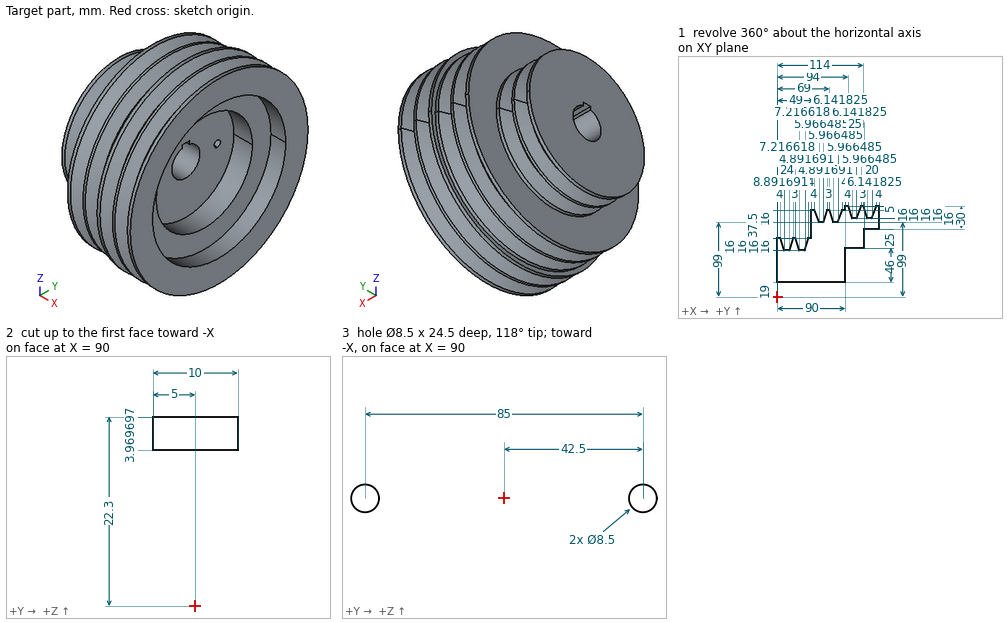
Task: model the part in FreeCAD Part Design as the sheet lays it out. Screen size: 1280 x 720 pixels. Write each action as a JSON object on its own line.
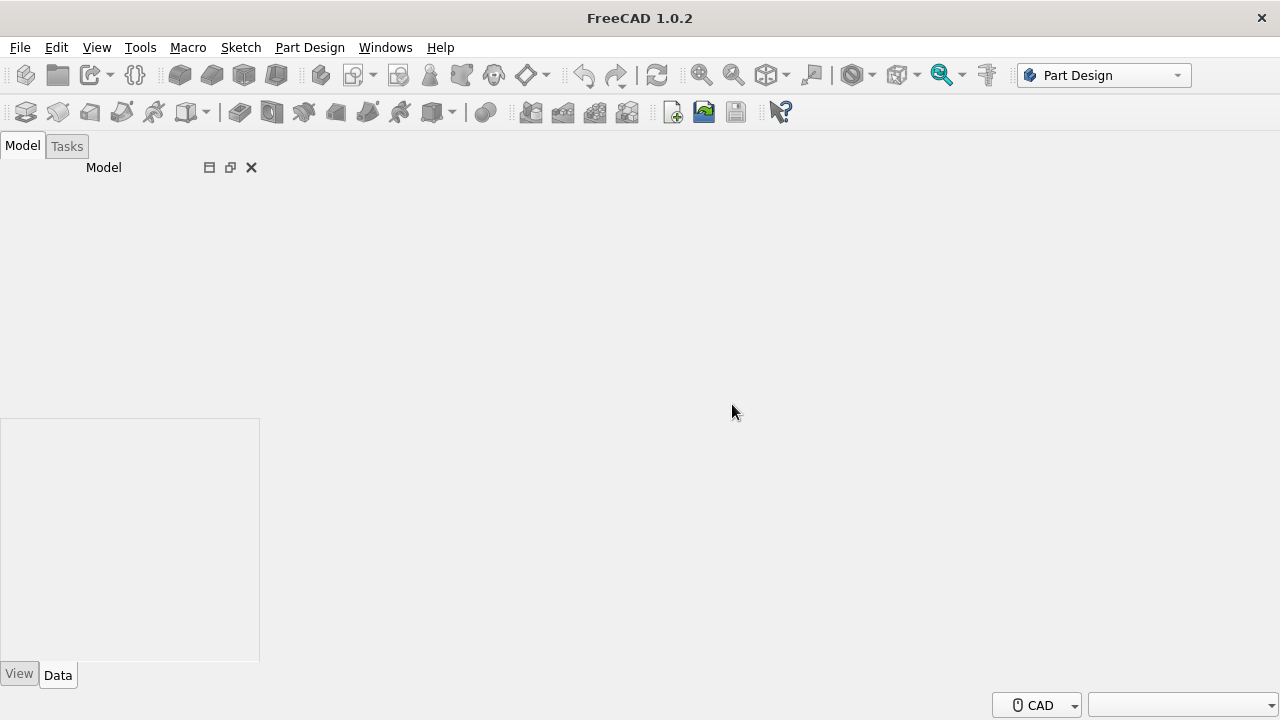
{"action": "key", "text": "ctrl+n"}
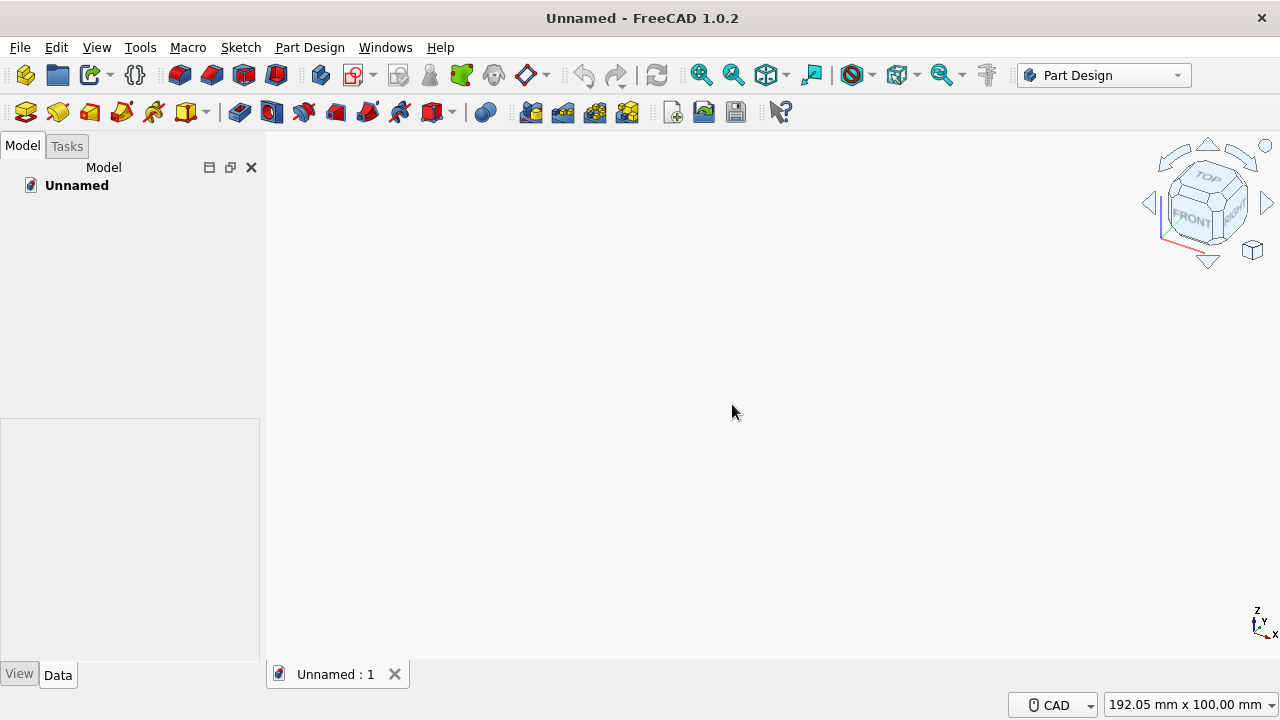
{"action": "left_click", "coordinate": [354, 76]}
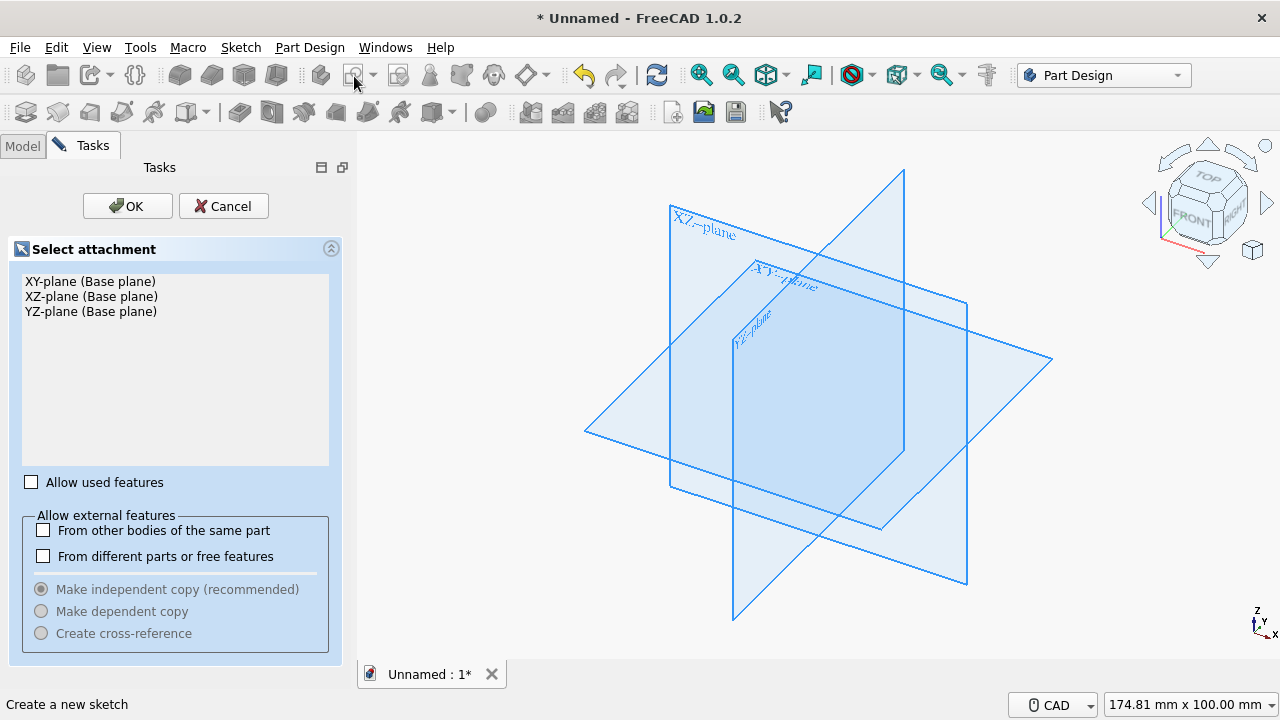
{"action": "left_click", "coordinate": [82, 282]}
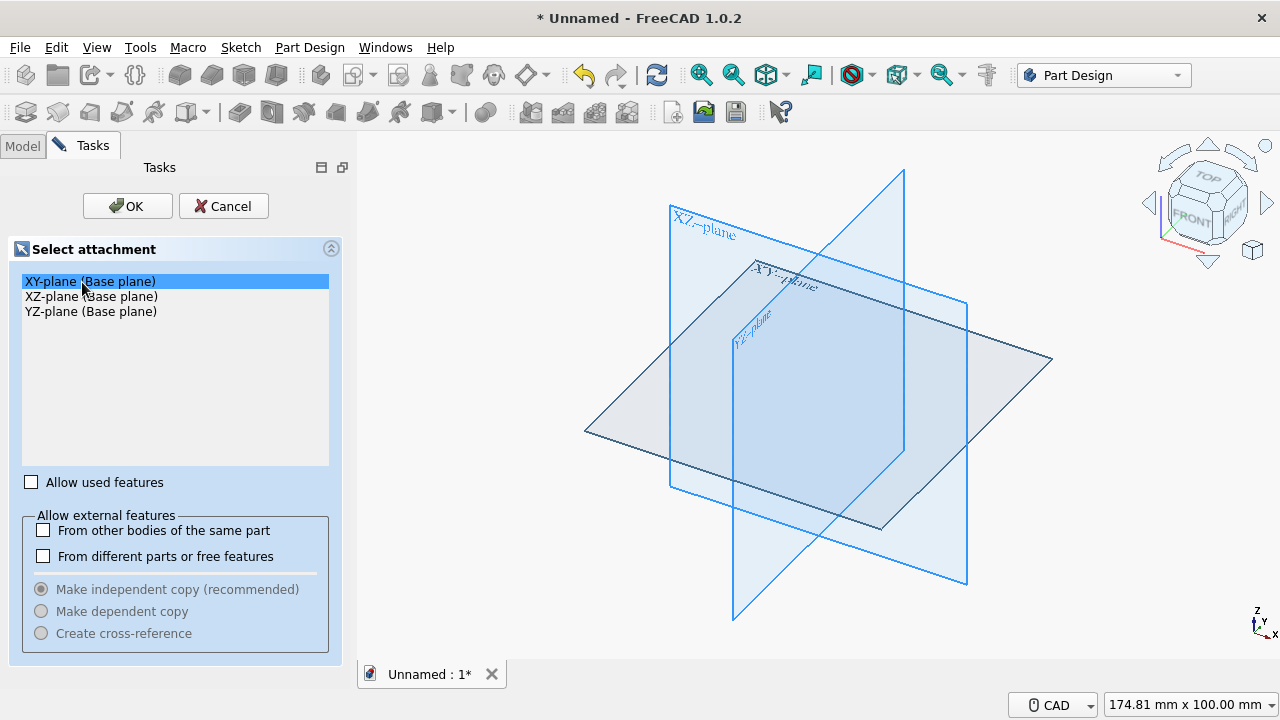
{"action": "left_click", "coordinate": [128, 206]}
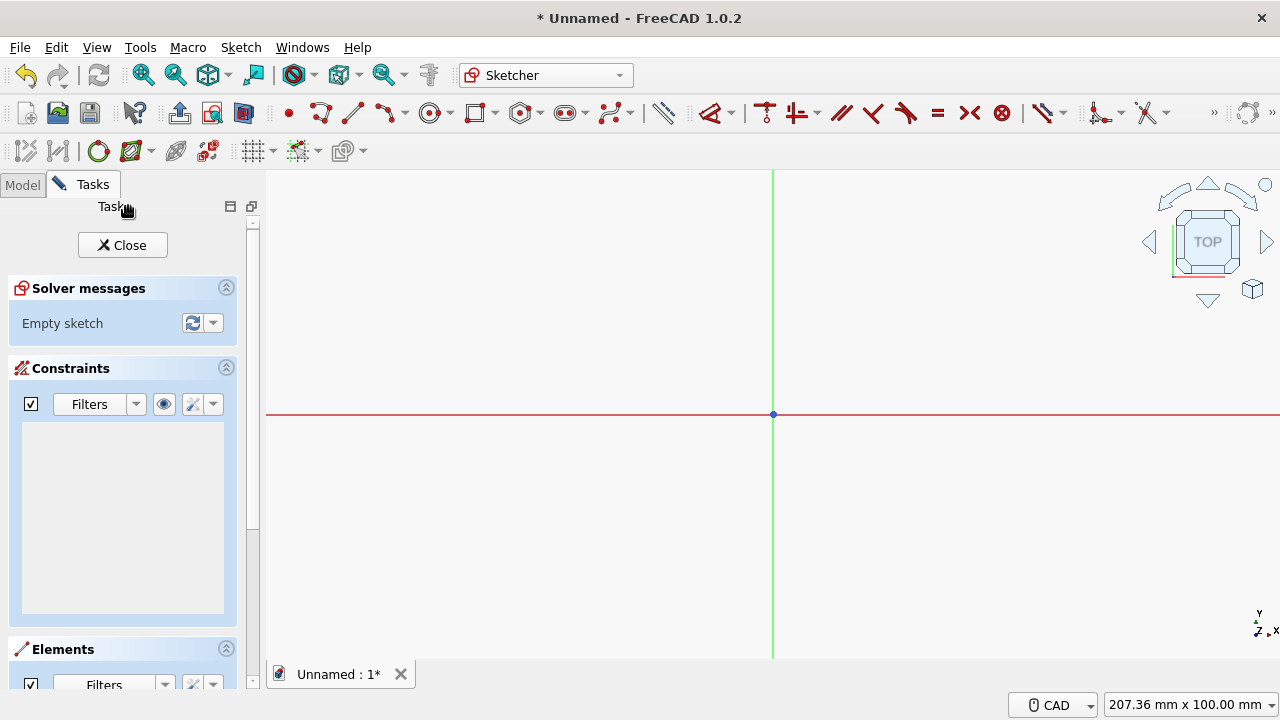
{"action": "scroll", "coordinate": [379, 631], "scroll_direction": "down", "scroll_amount": 4}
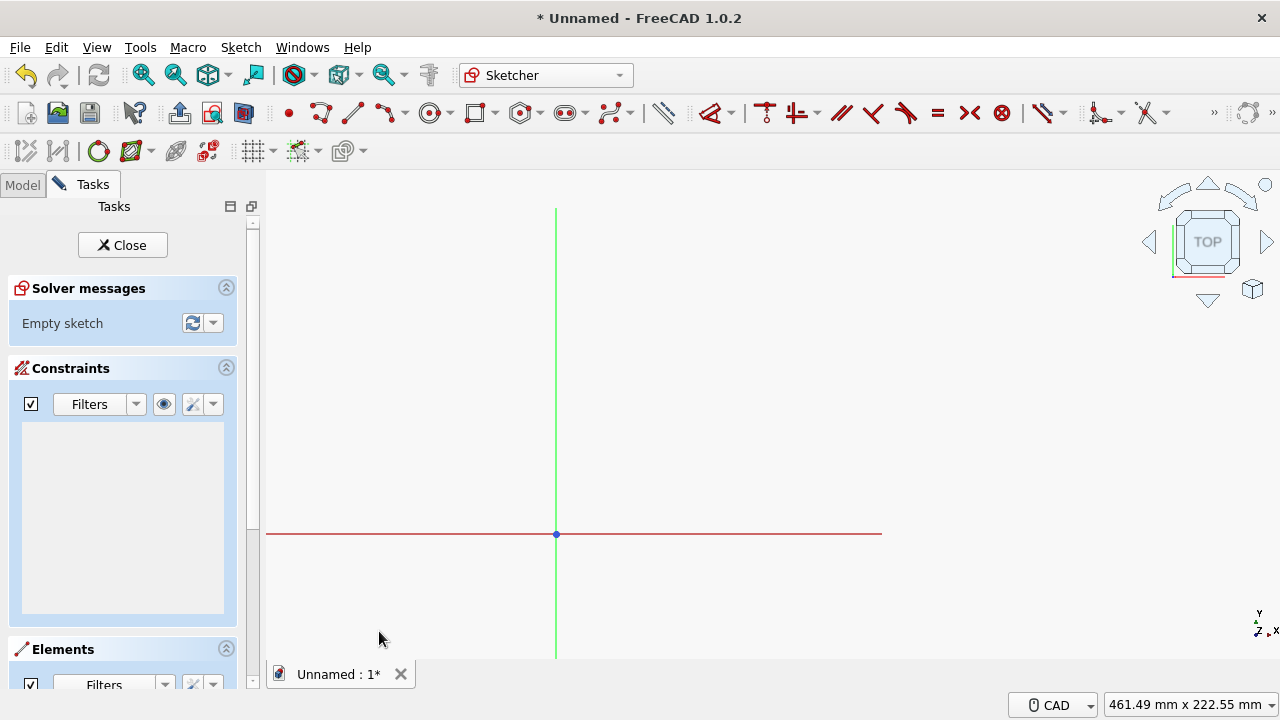
{"action": "key", "text": "g m"}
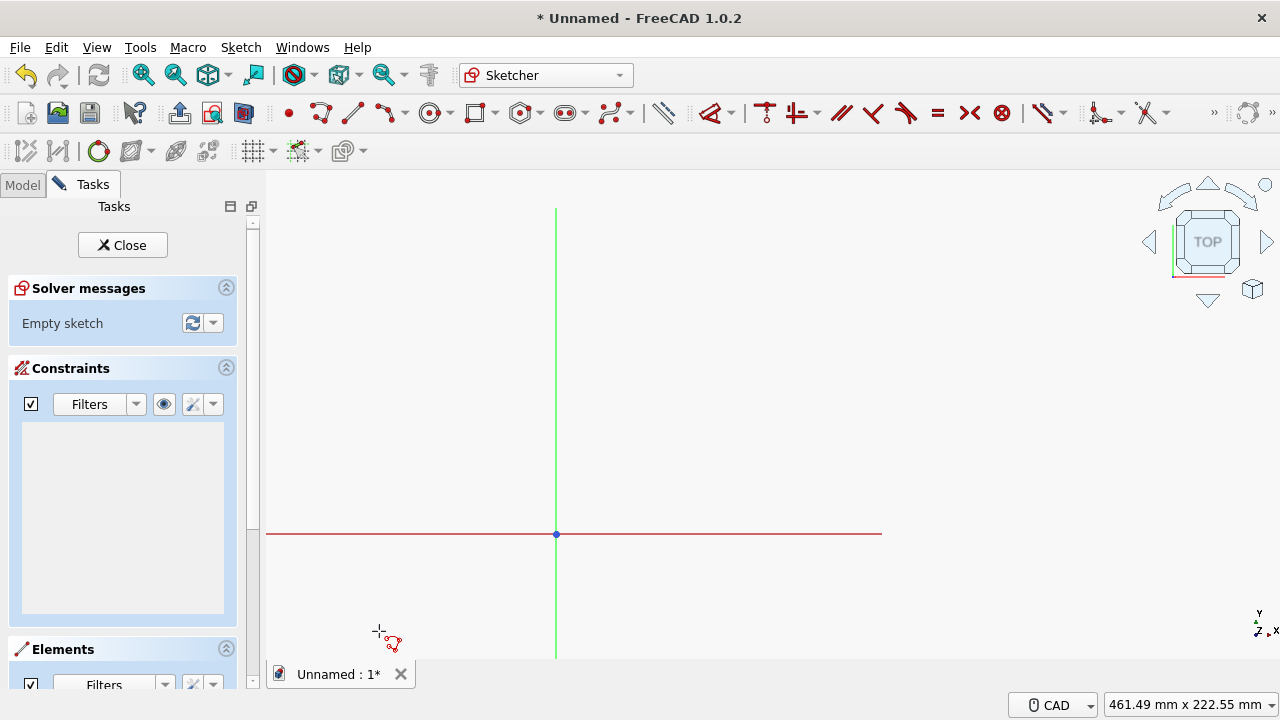
{"action": "left_click", "coordinate": [556, 492]}
{"action": "left_click", "coordinate": [754, 492]}
{"action": "left_click", "coordinate": [754, 391]}
{"action": "left_click", "coordinate": [809, 391]}
{"action": "left_click", "coordinate": [809, 336]}
{"action": "left_click", "coordinate": [853, 336]}
{"action": "left_click", "coordinate": [853, 271]}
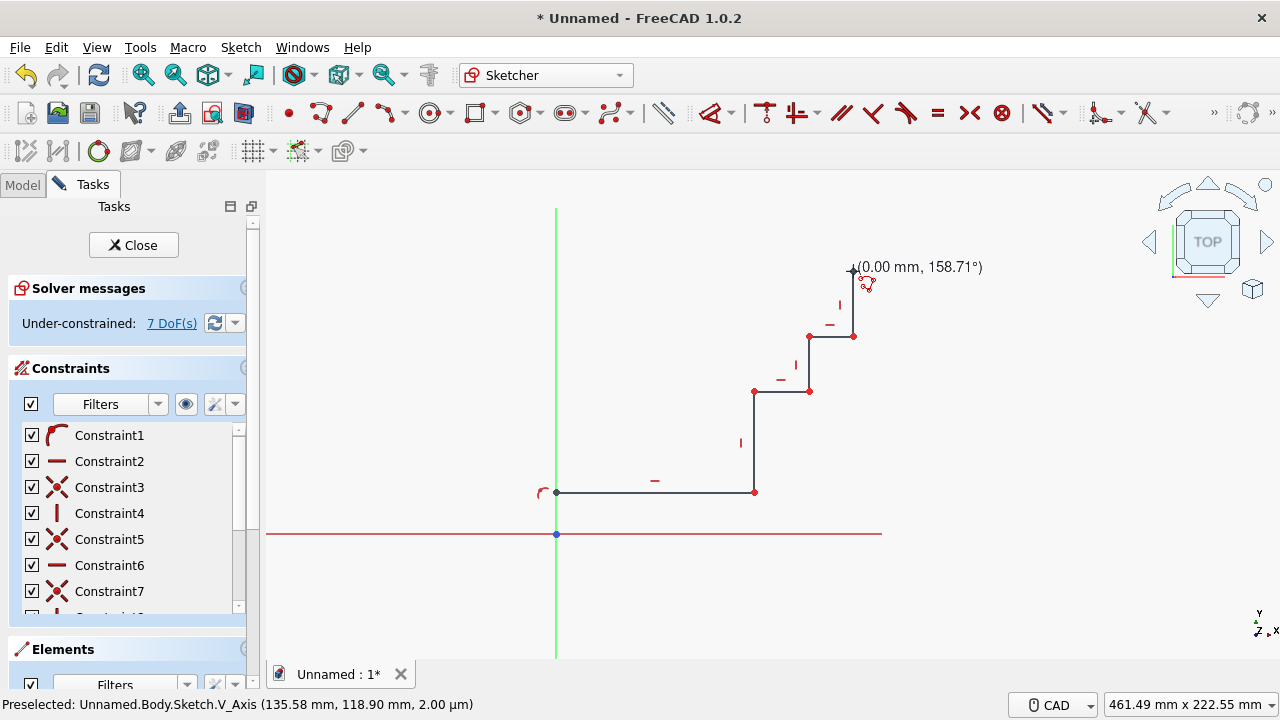
{"action": "scroll", "coordinate": [844, 271], "scroll_direction": "up", "scroll_amount": 3}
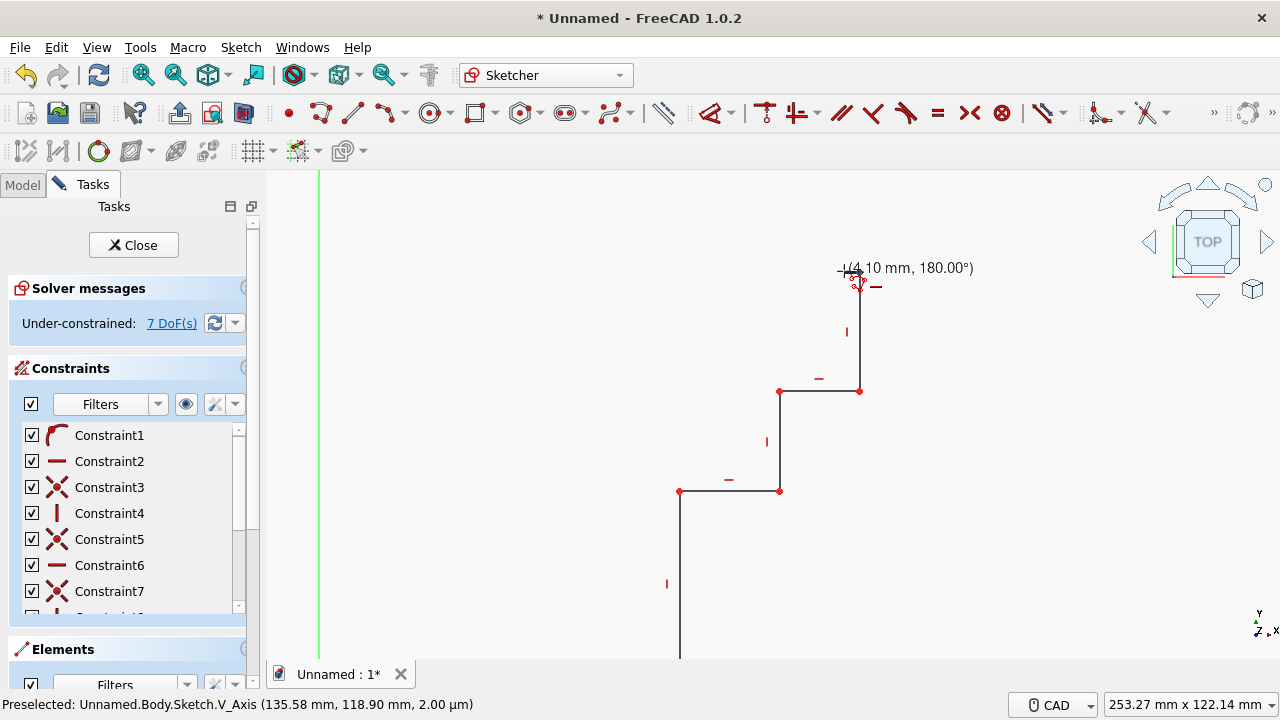
{"action": "left_click", "coordinate": [843, 271]}
{"action": "left_click", "coordinate": [819, 334]}
{"action": "left_click", "coordinate": [795, 334]}
{"action": "left_click", "coordinate": [775, 270]}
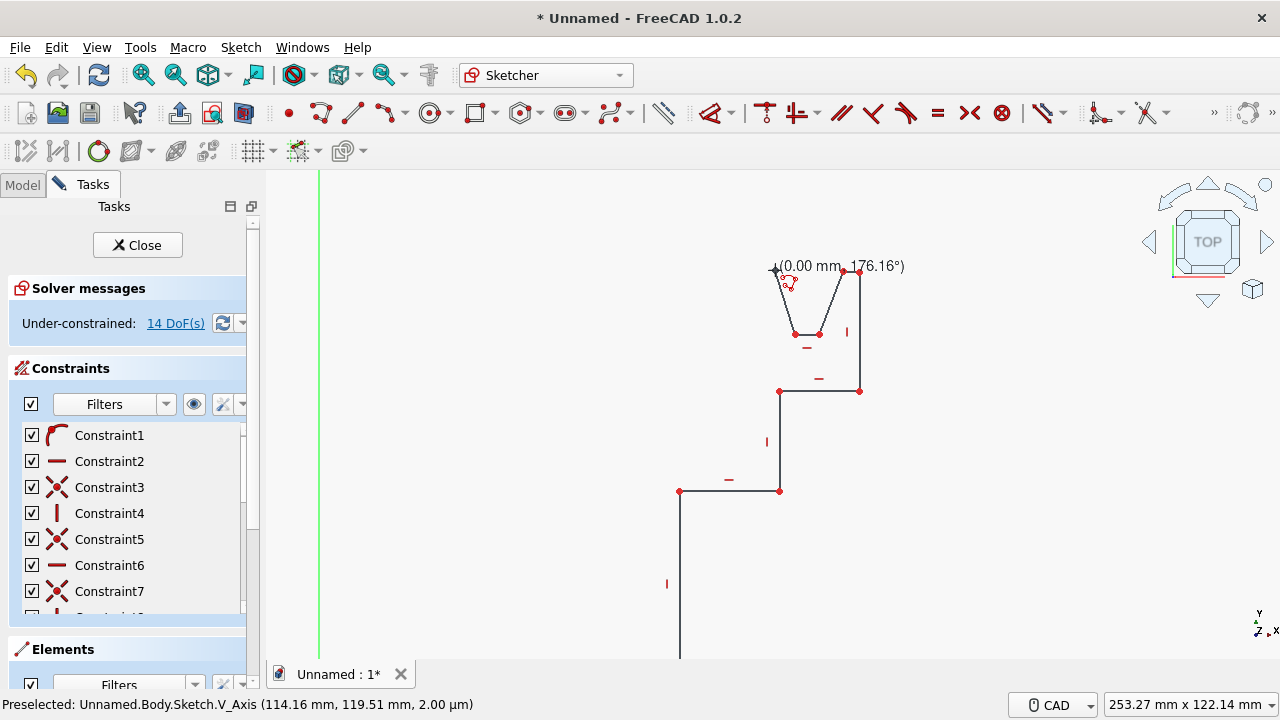
{"action": "scroll", "coordinate": [763, 270], "scroll_direction": "up", "scroll_amount": 2}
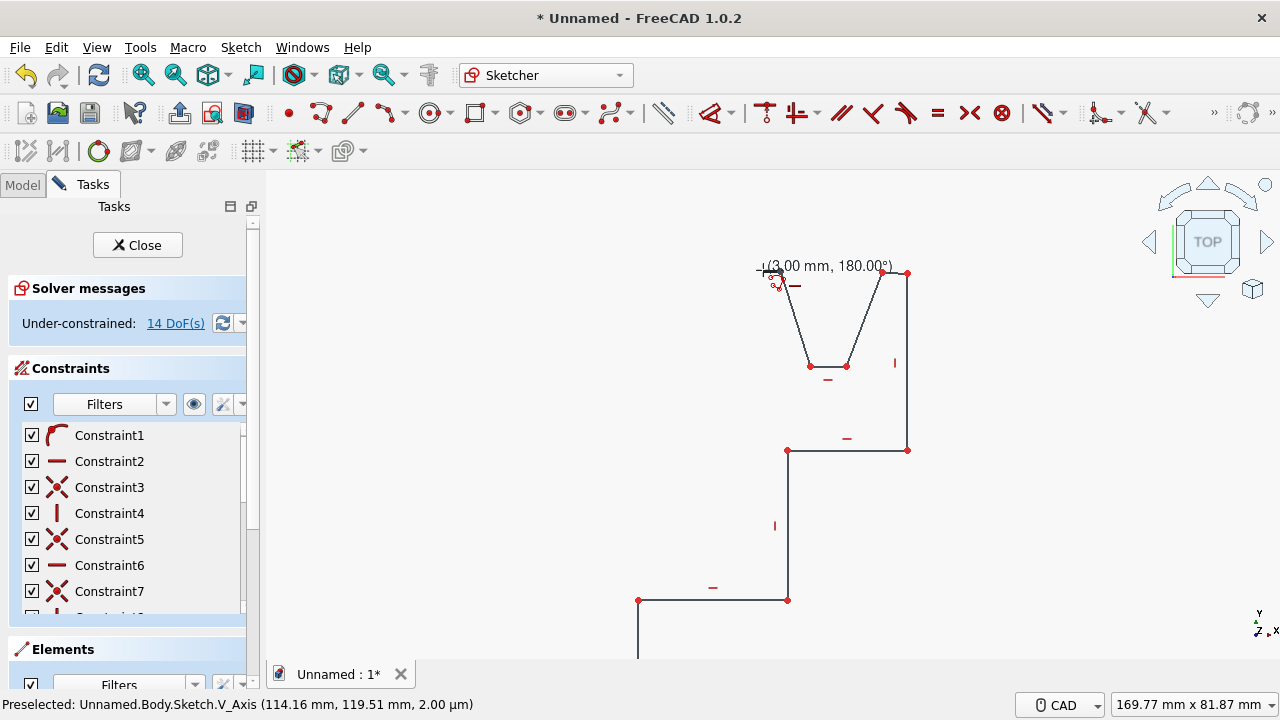
{"action": "left_click", "coordinate": [763, 270]}
{"action": "left_click", "coordinate": [727, 366]}
{"action": "left_click", "coordinate": [691, 366]}
{"action": "left_click", "coordinate": [662, 270]}
{"action": "left_click", "coordinate": [638, 270]}
{"action": "left_click", "coordinate": [638, 300]}
{"action": "left_click", "coordinate": [614, 300]}
{"action": "left_click", "coordinate": [577, 395]}
{"action": "left_click", "coordinate": [542, 395]}
{"action": "left_click", "coordinate": [512, 300]}
{"action": "left_click", "coordinate": [494, 300]}
{"action": "left_click", "coordinate": [465, 395]}
{"action": "left_click", "coordinate": [430, 395]}
{"action": "left_click", "coordinate": [393, 300]}
{"action": "left_click", "coordinate": [369, 300]}
{"action": "left_click", "coordinate": [369, 524]}
{"action": "left_click", "coordinate": [345, 524]}
{"action": "left_click", "coordinate": [316, 619]}